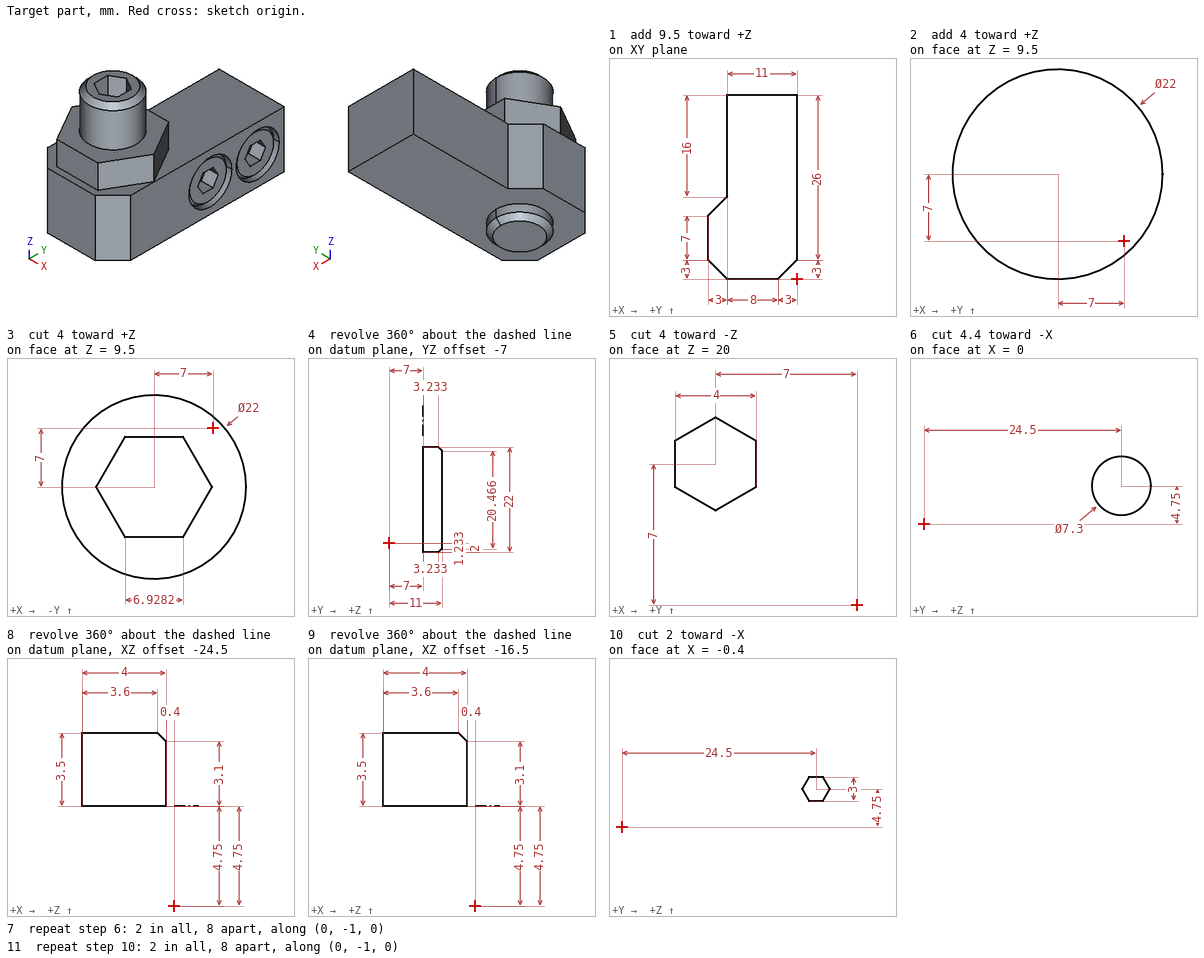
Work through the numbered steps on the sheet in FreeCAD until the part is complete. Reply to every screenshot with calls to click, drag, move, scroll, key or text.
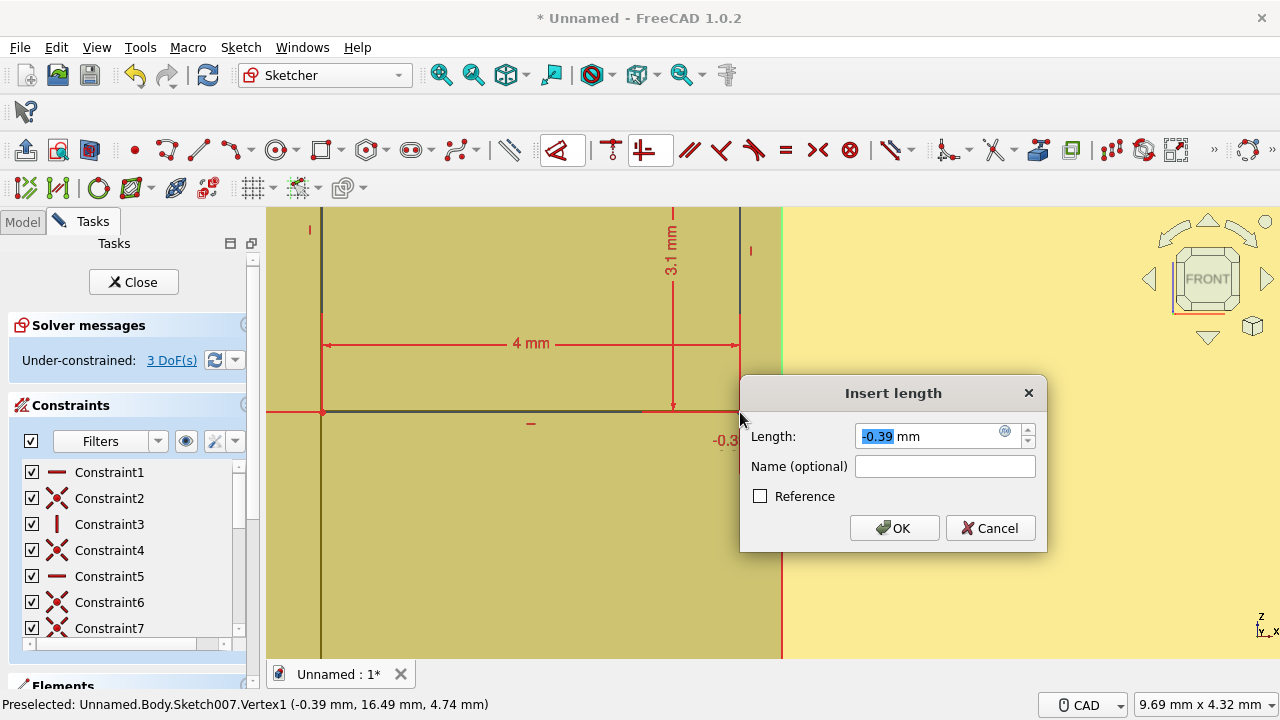
text(-0.4)
key(Return)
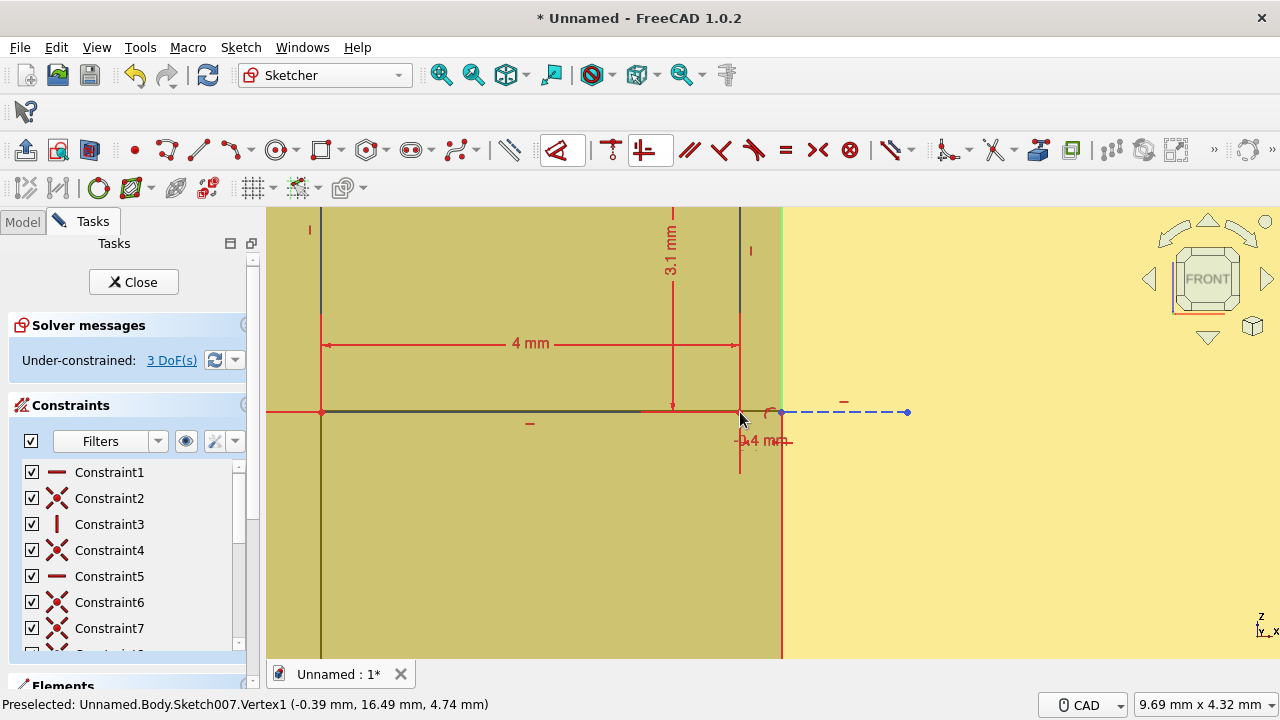
click(740, 412)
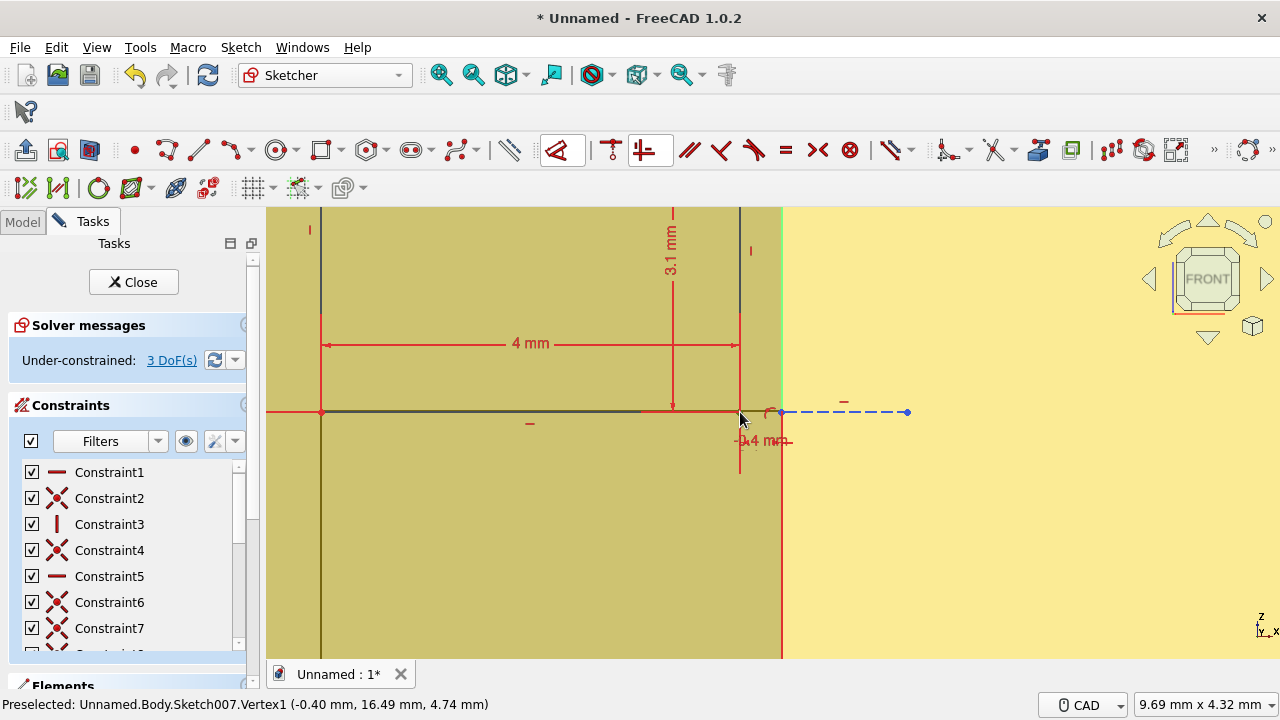
key(i)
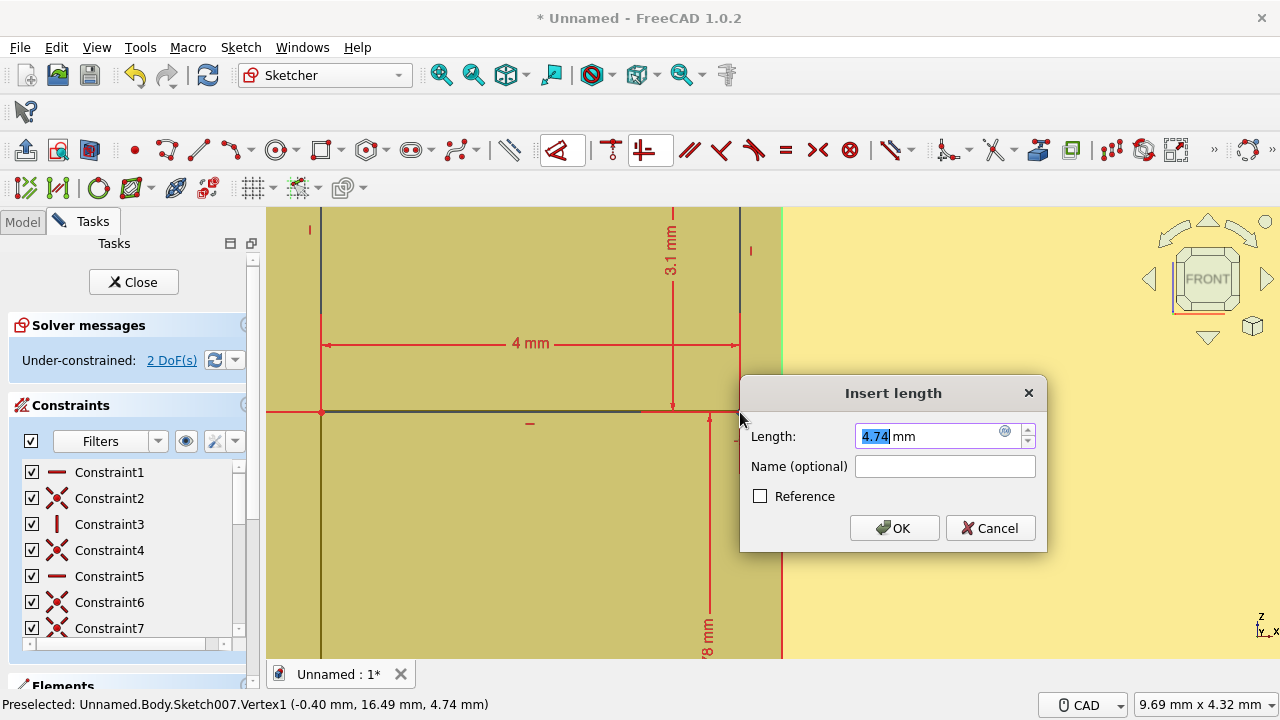
text(4.75)
key(Return)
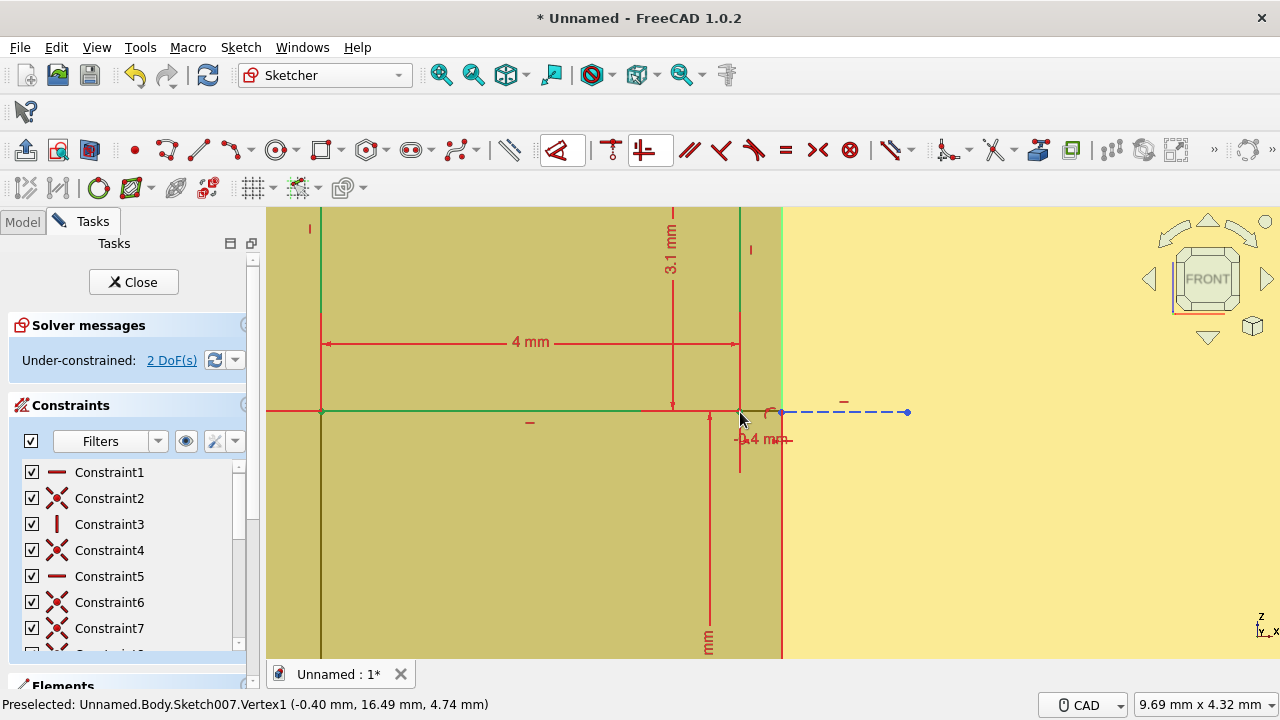
click(782, 412)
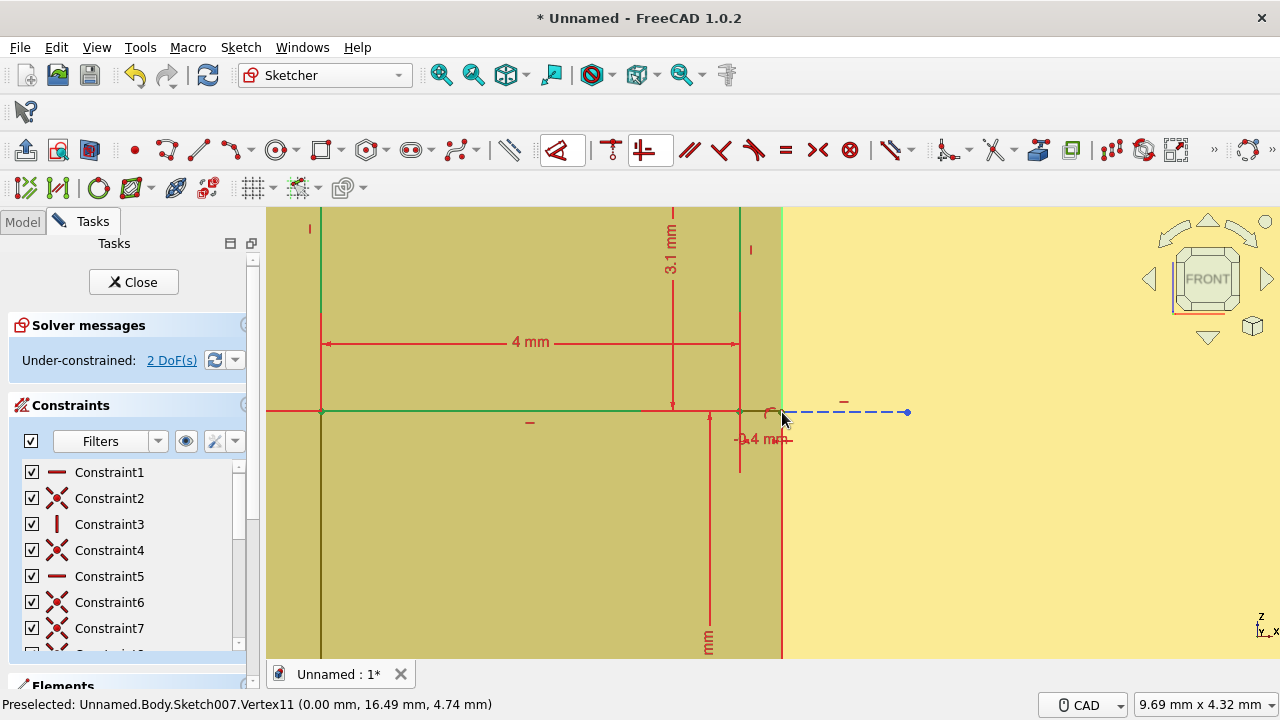
key(i)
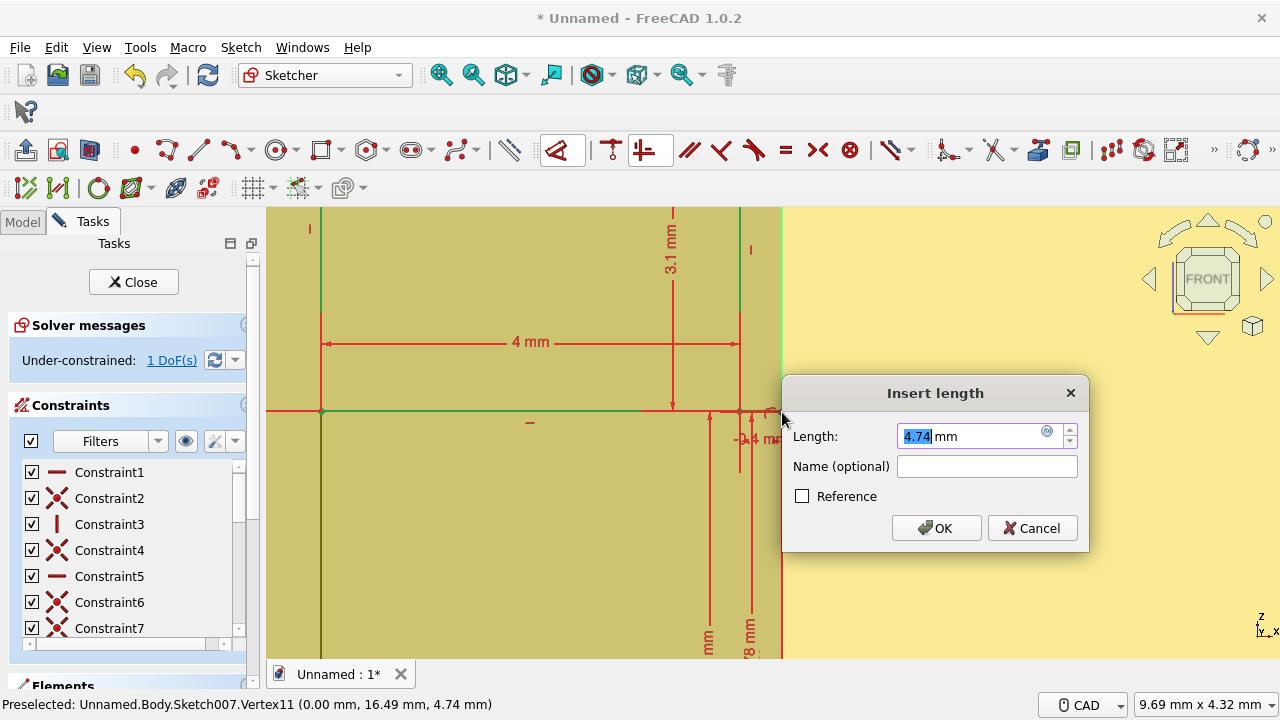
text(4.75)
key(Return)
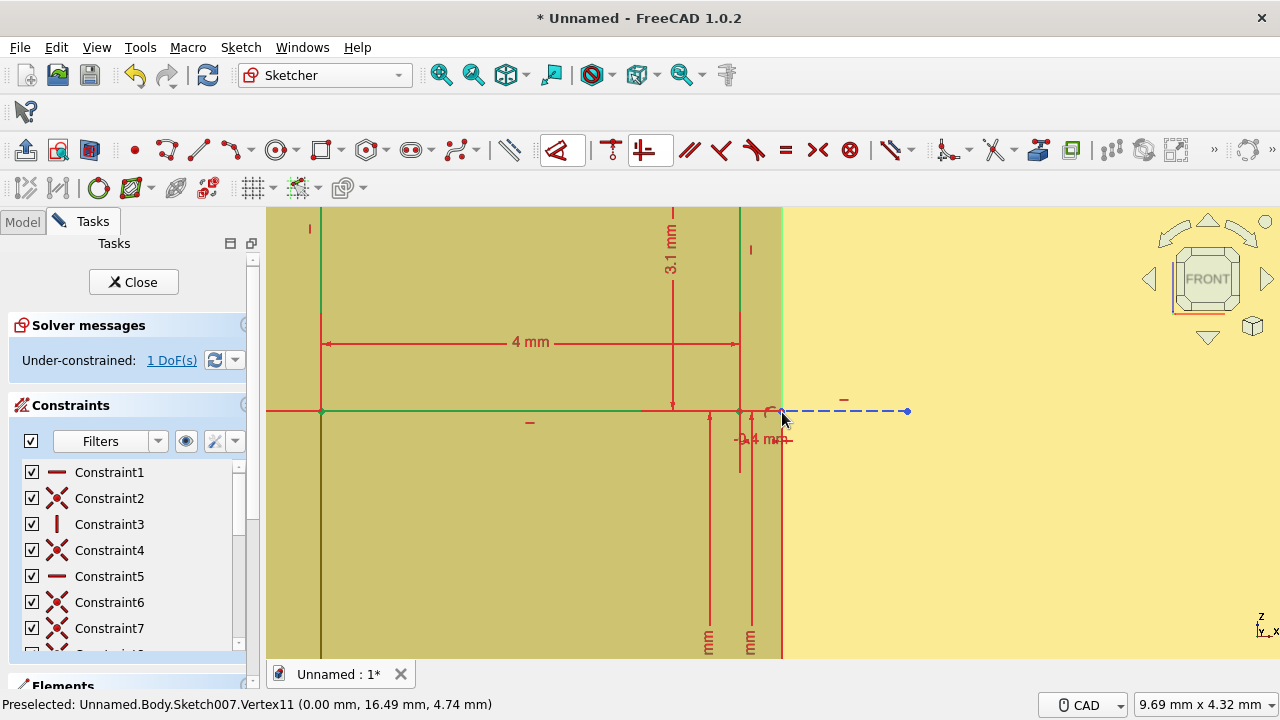
click(134, 282)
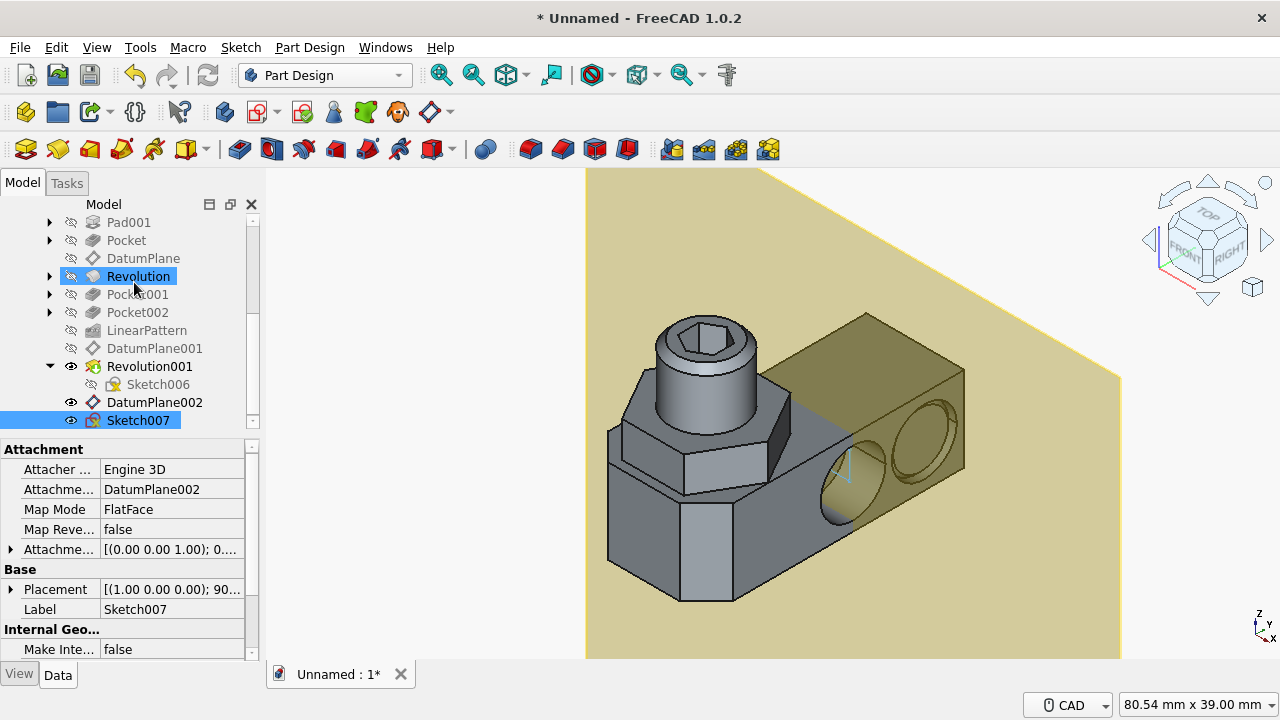
click(58, 150)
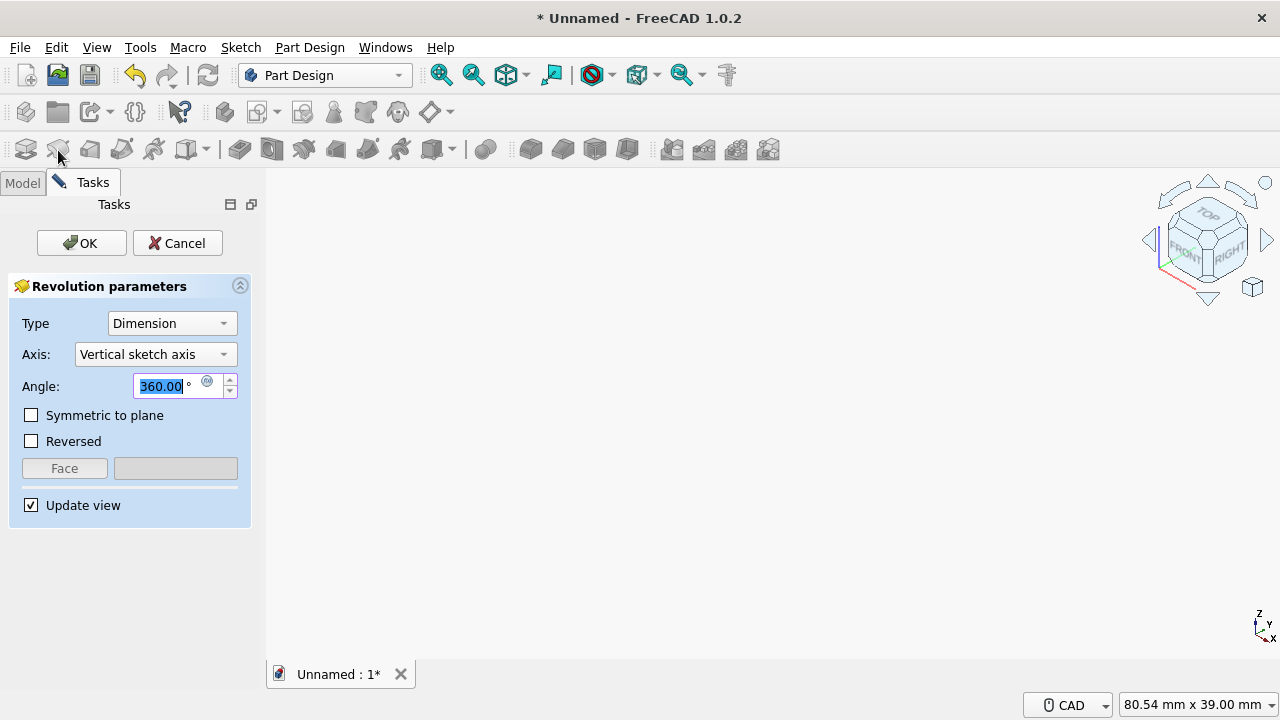
click(156, 354)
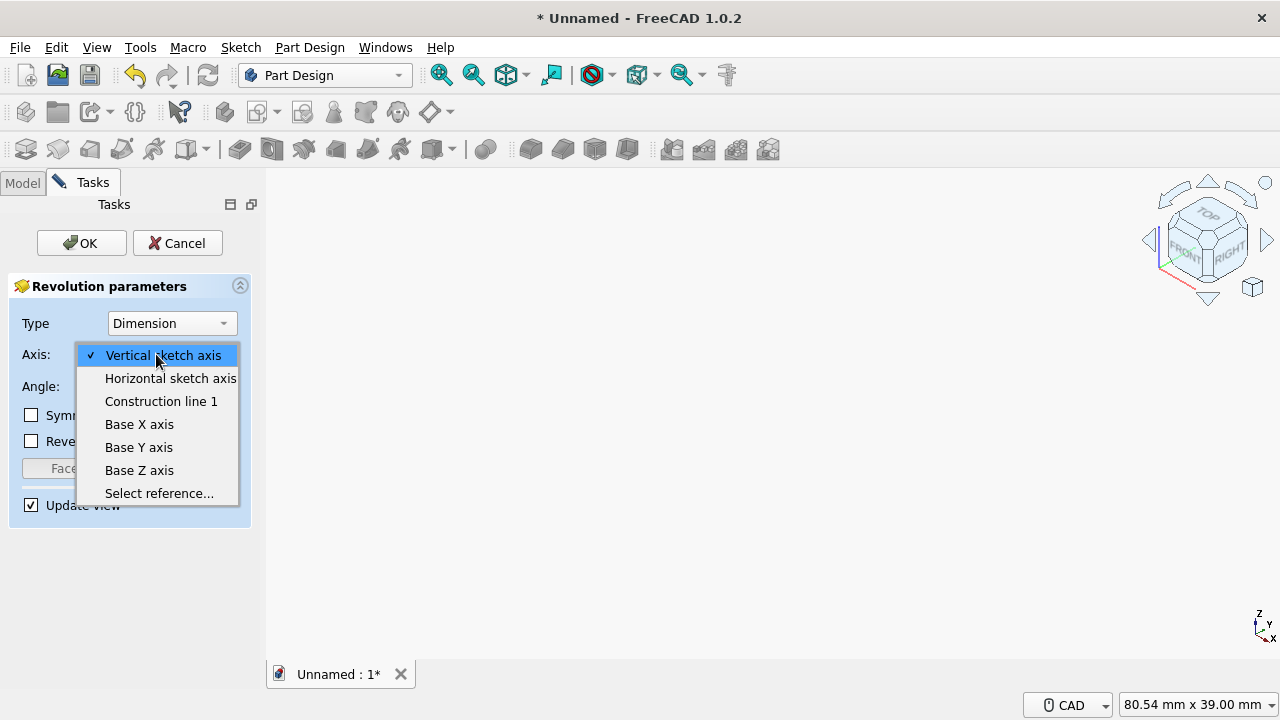
click(156, 402)